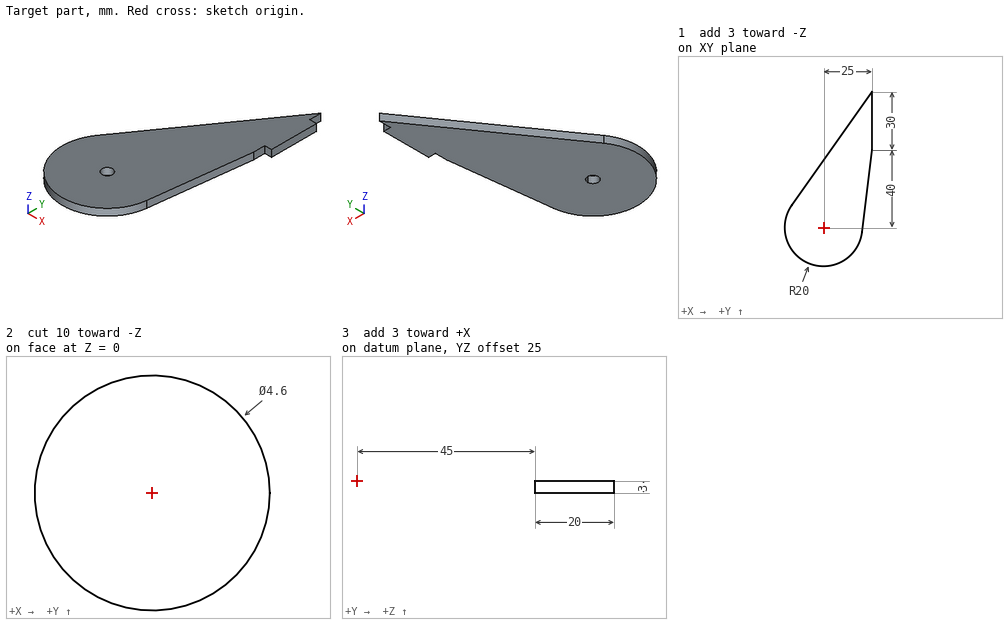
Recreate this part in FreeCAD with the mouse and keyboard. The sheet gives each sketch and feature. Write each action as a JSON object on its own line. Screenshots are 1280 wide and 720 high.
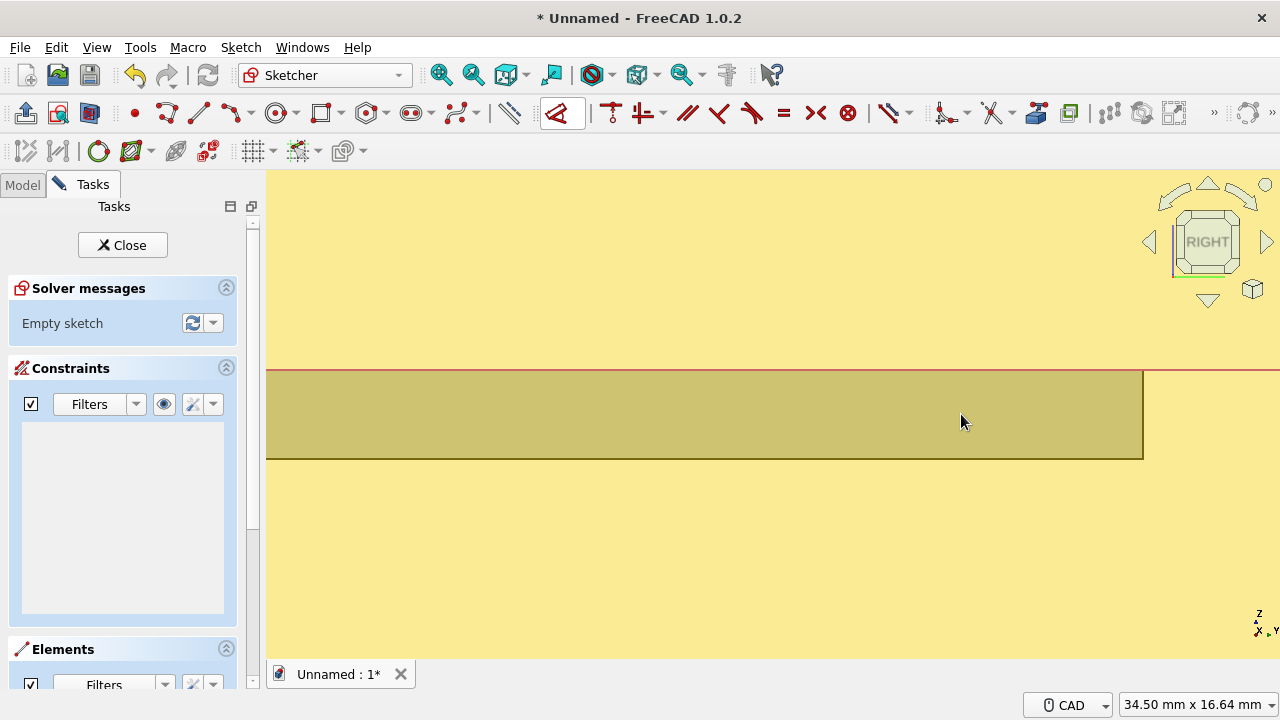
{"action": "left_click", "coordinate": [322, 114]}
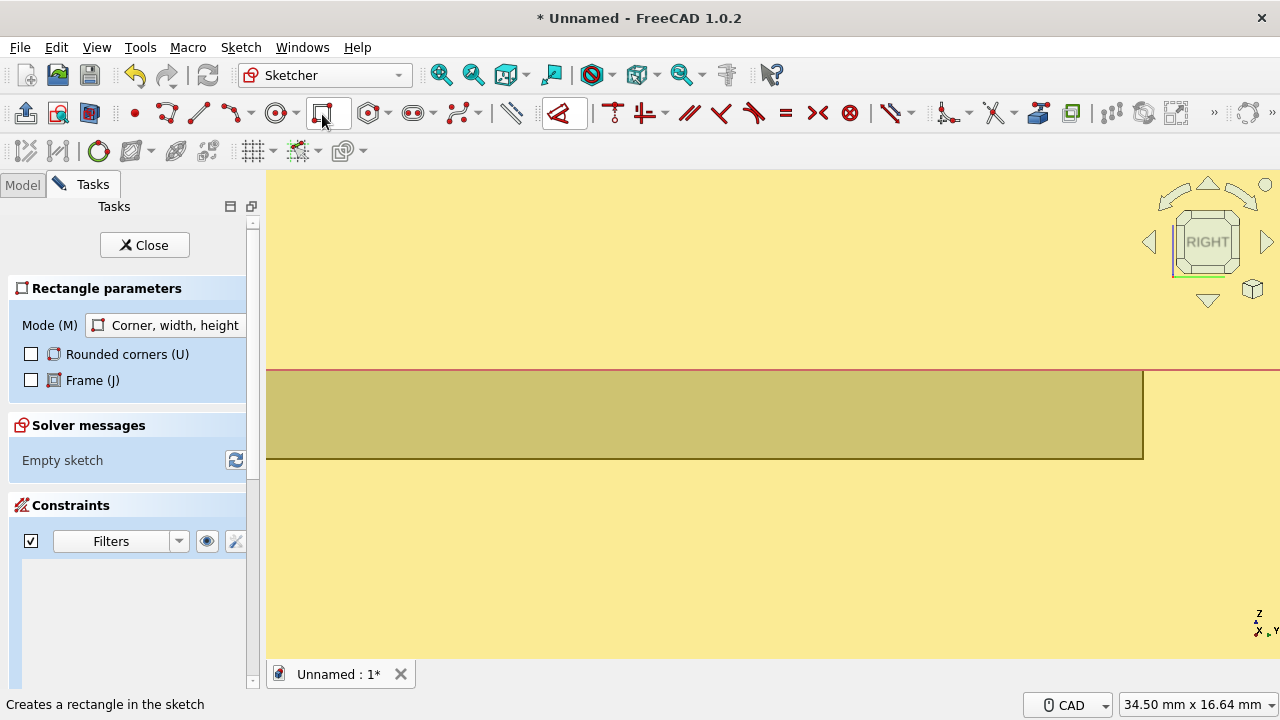
{"action": "left_click", "coordinate": [408, 370]}
{"action": "mouse_move", "coordinate": [996, 459]}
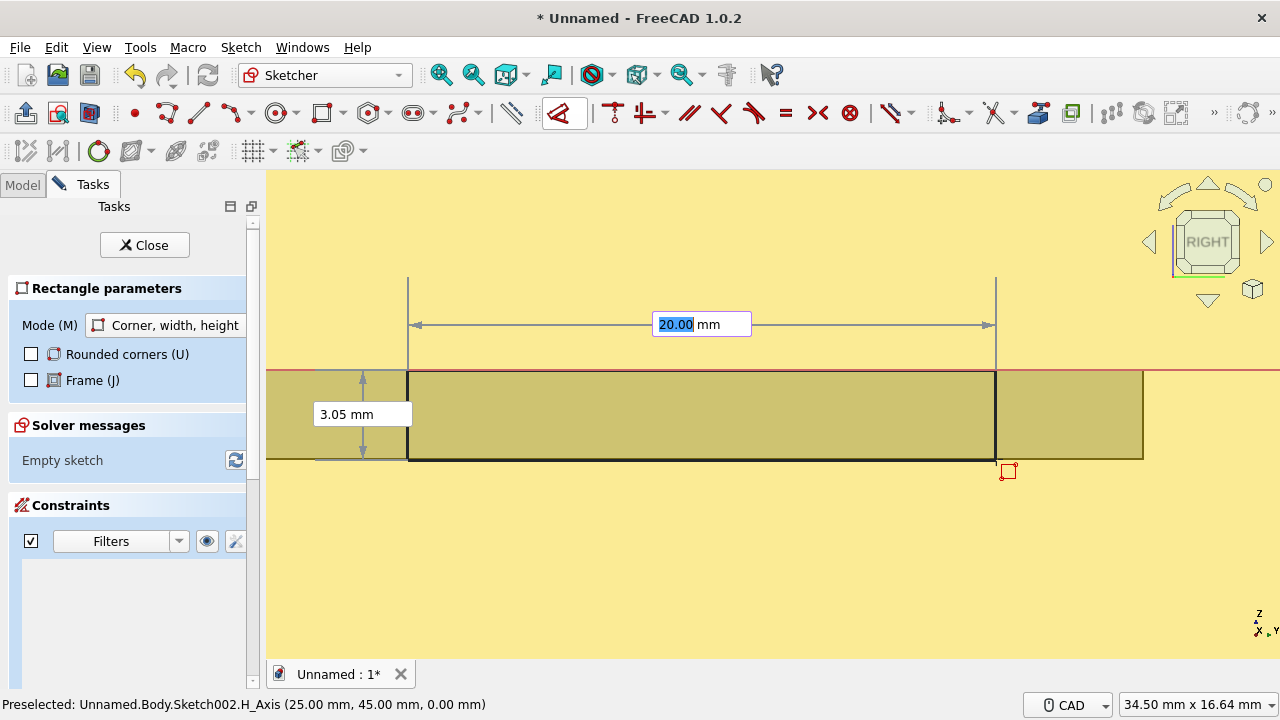
{"action": "type", "text": "20"}
{"action": "key", "text": "Tab"}
{"action": "type", "text": "3"}
{"action": "key", "text": "Return"}
{"action": "key", "text": "Escape"}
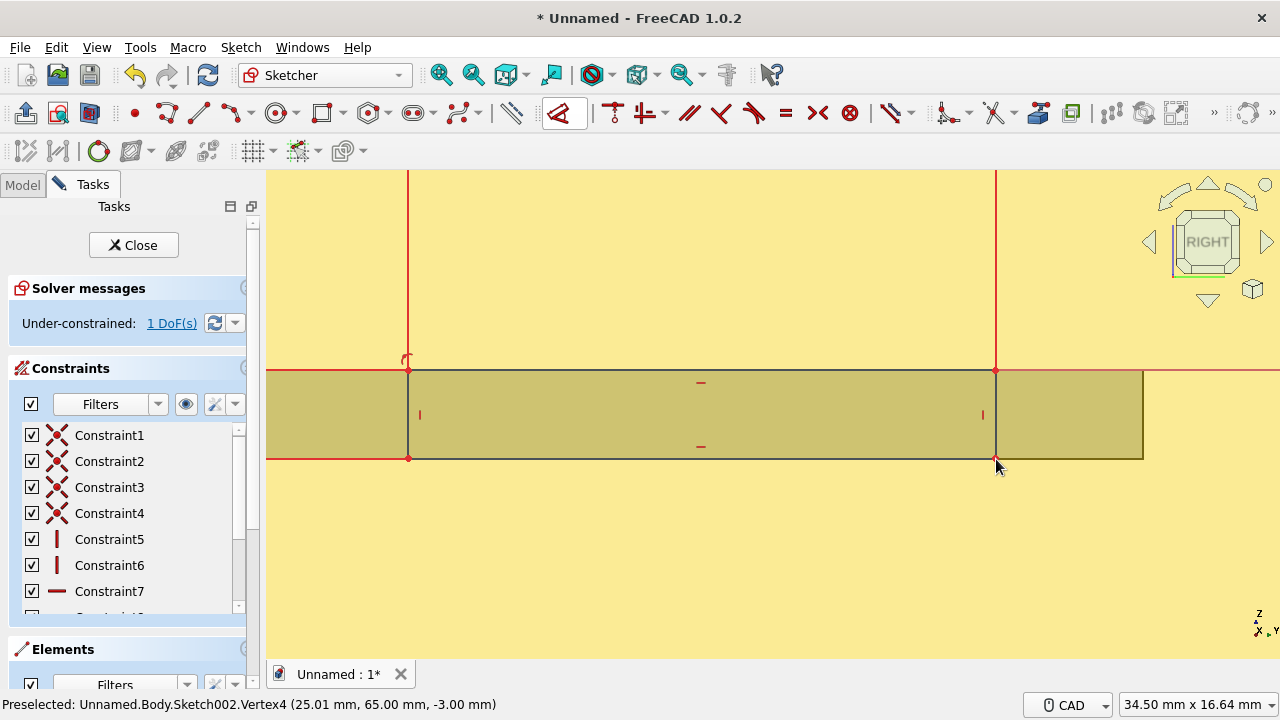
{"action": "left_click", "coordinate": [408, 370]}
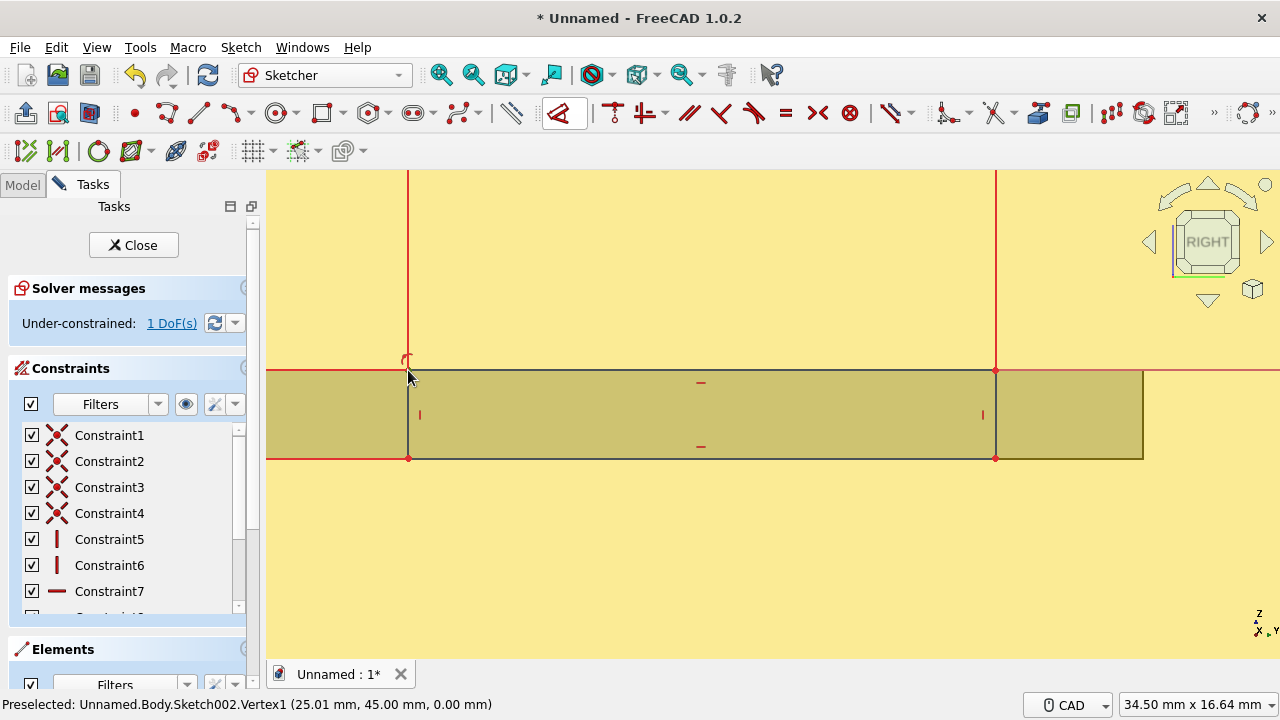
{"action": "key", "text": "l"}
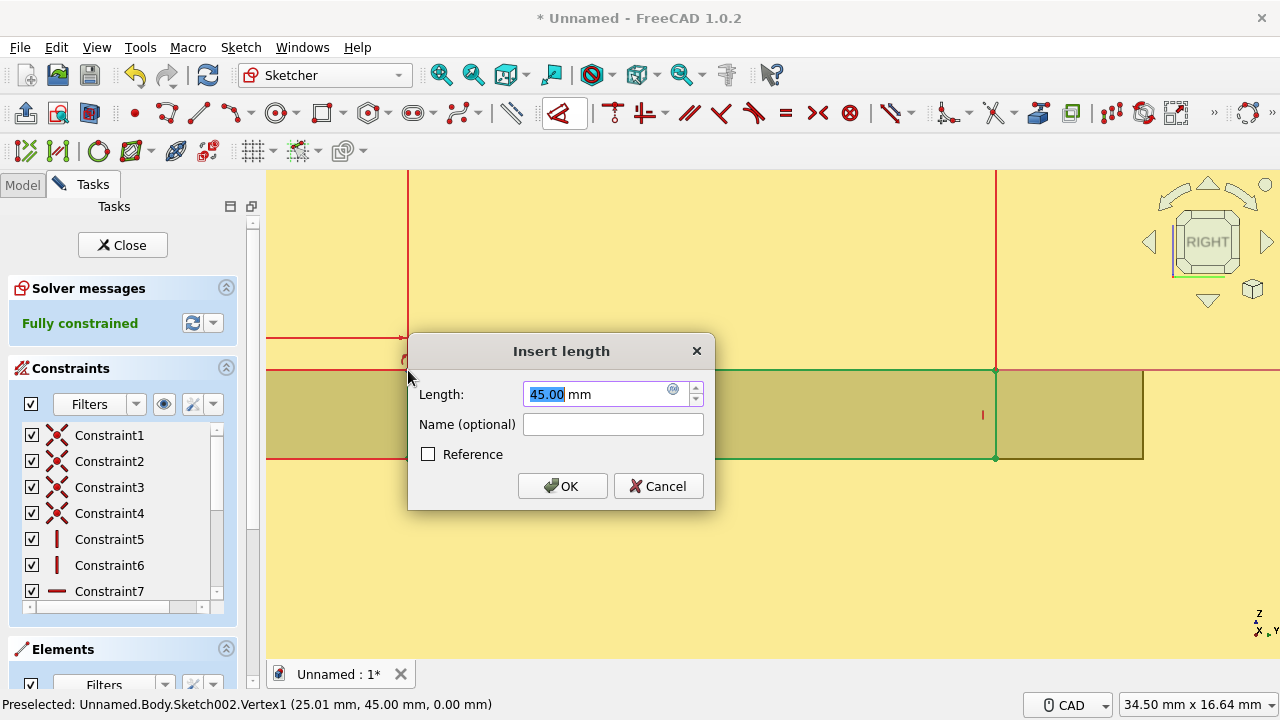
{"action": "type", "text": "45"}
{"action": "key", "text": "Return"}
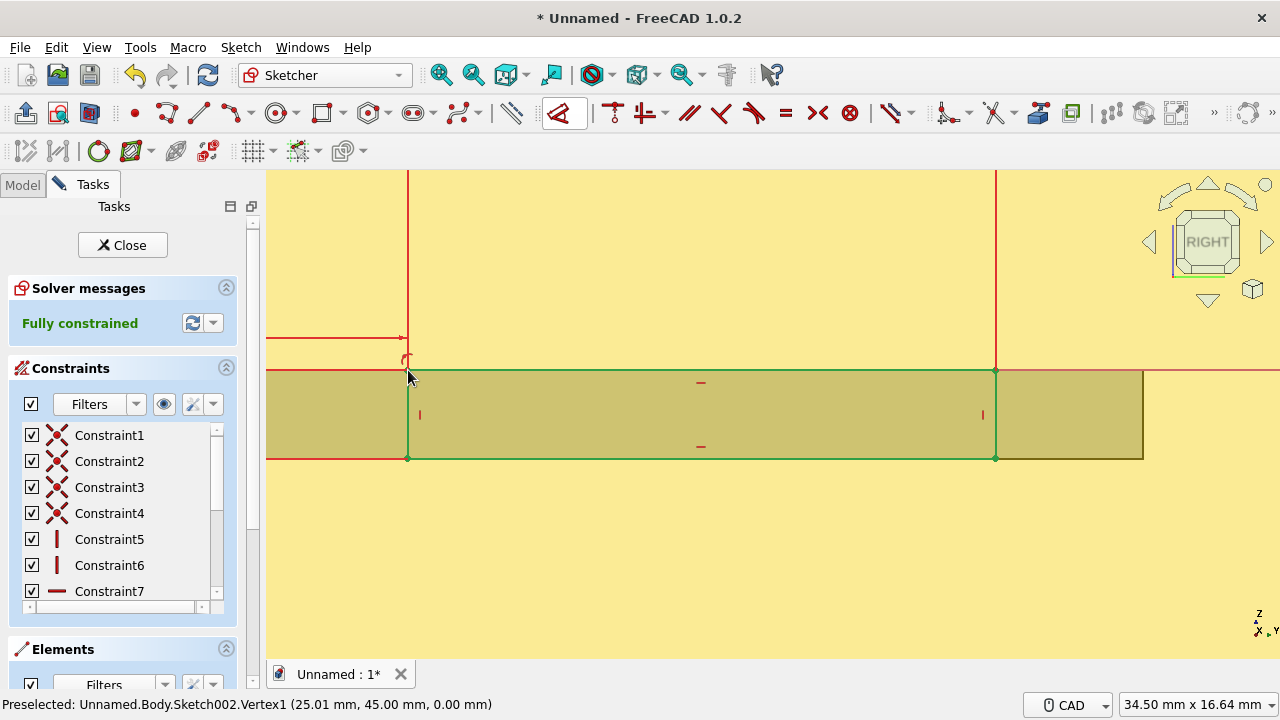
{"action": "left_click", "coordinate": [123, 245]}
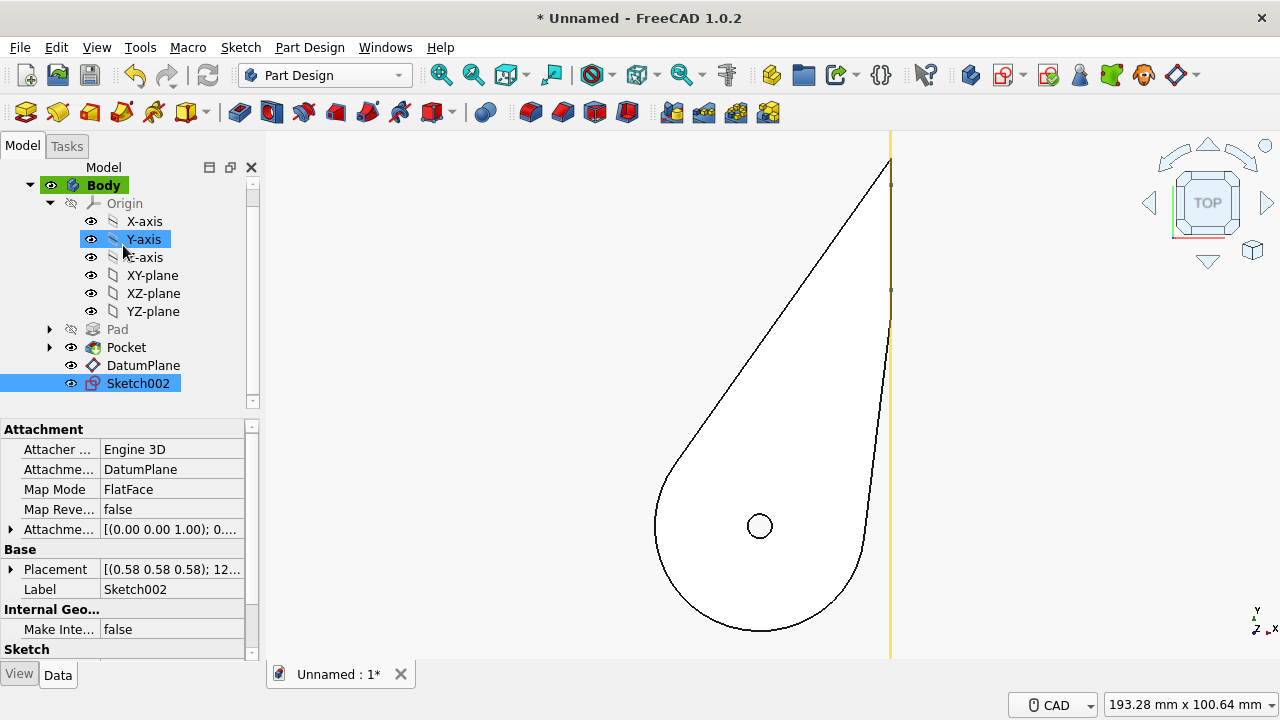
{"action": "left_click", "coordinate": [26, 112]}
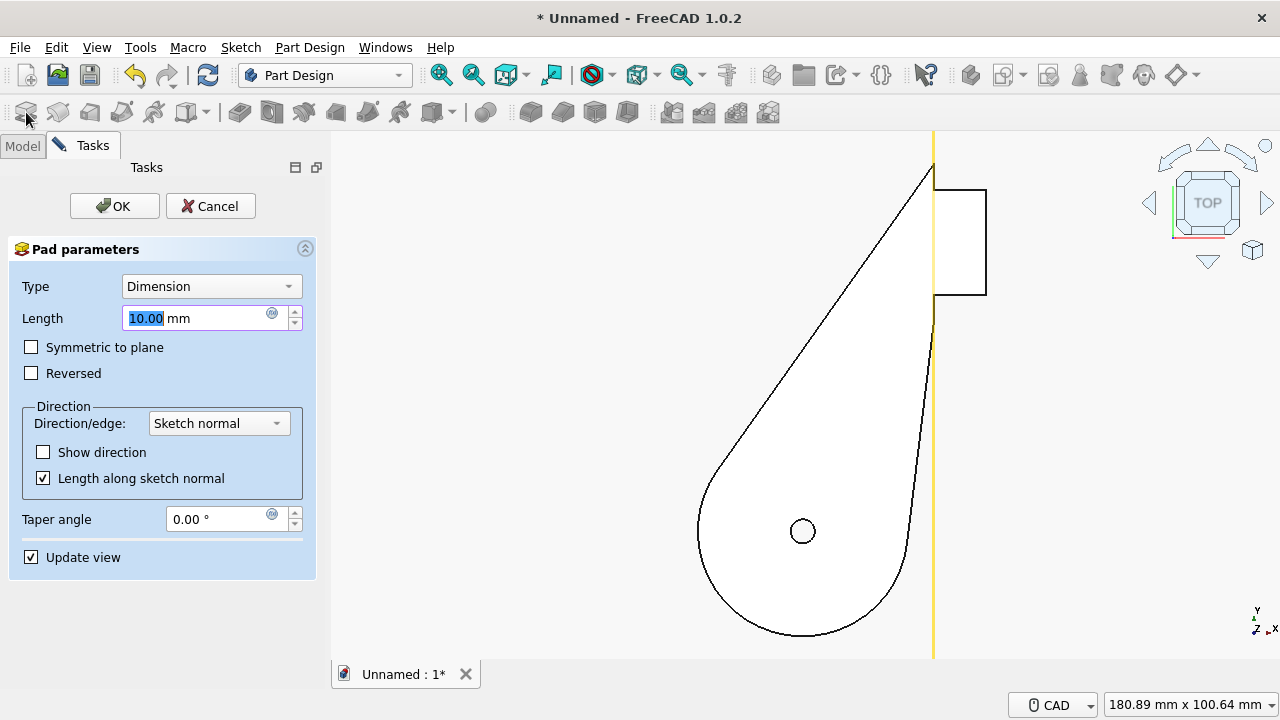
{"action": "type", "text": "3"}
{"action": "key", "text": "Tab"}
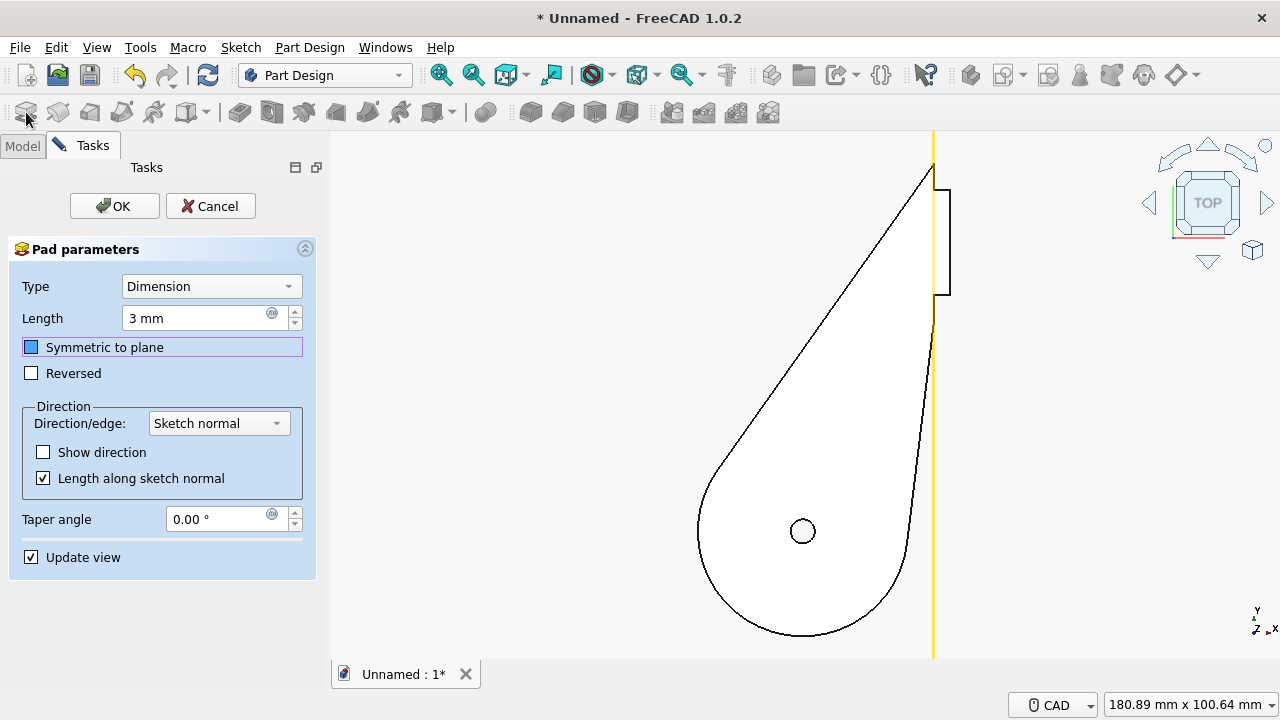
{"action": "left_click", "coordinate": [115, 206]}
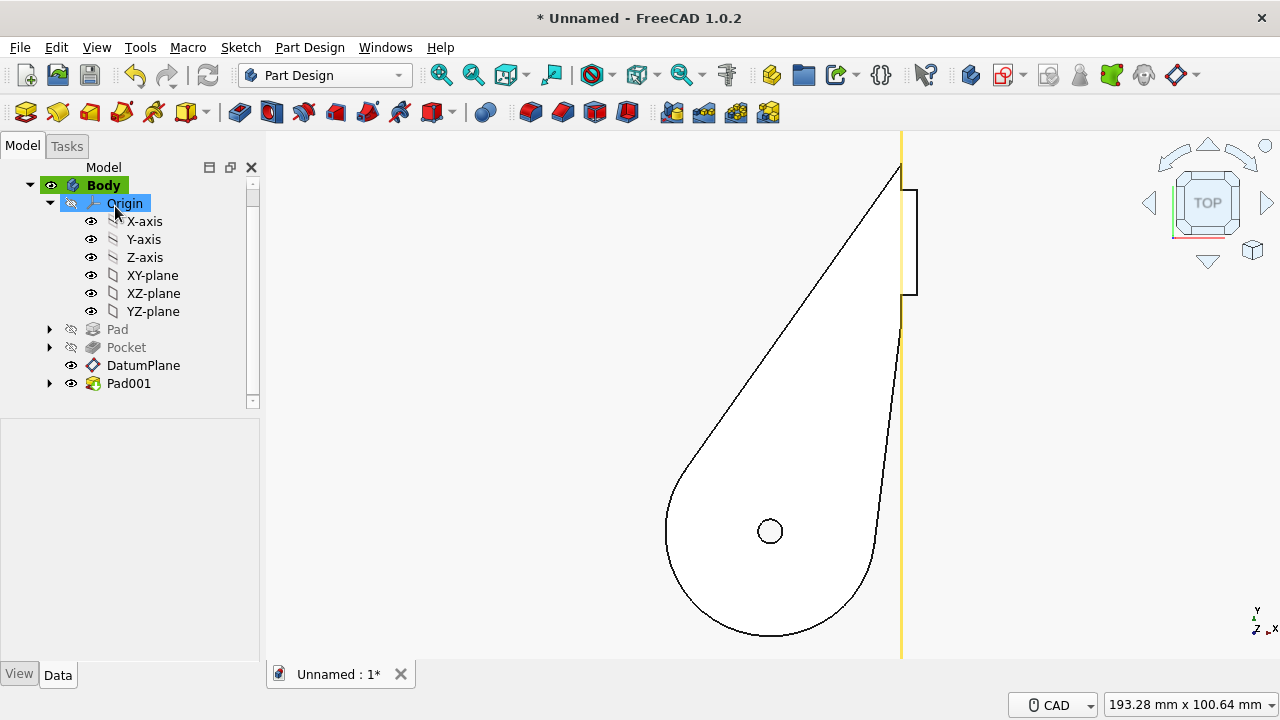
{"action": "left_click", "coordinate": [116, 365]}
{"action": "key", "text": "space"}